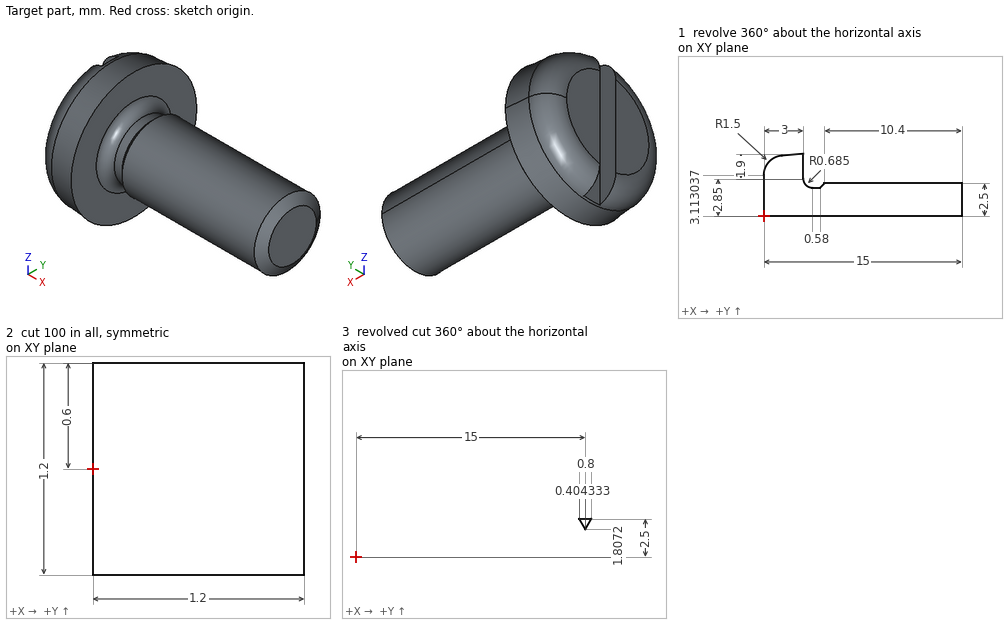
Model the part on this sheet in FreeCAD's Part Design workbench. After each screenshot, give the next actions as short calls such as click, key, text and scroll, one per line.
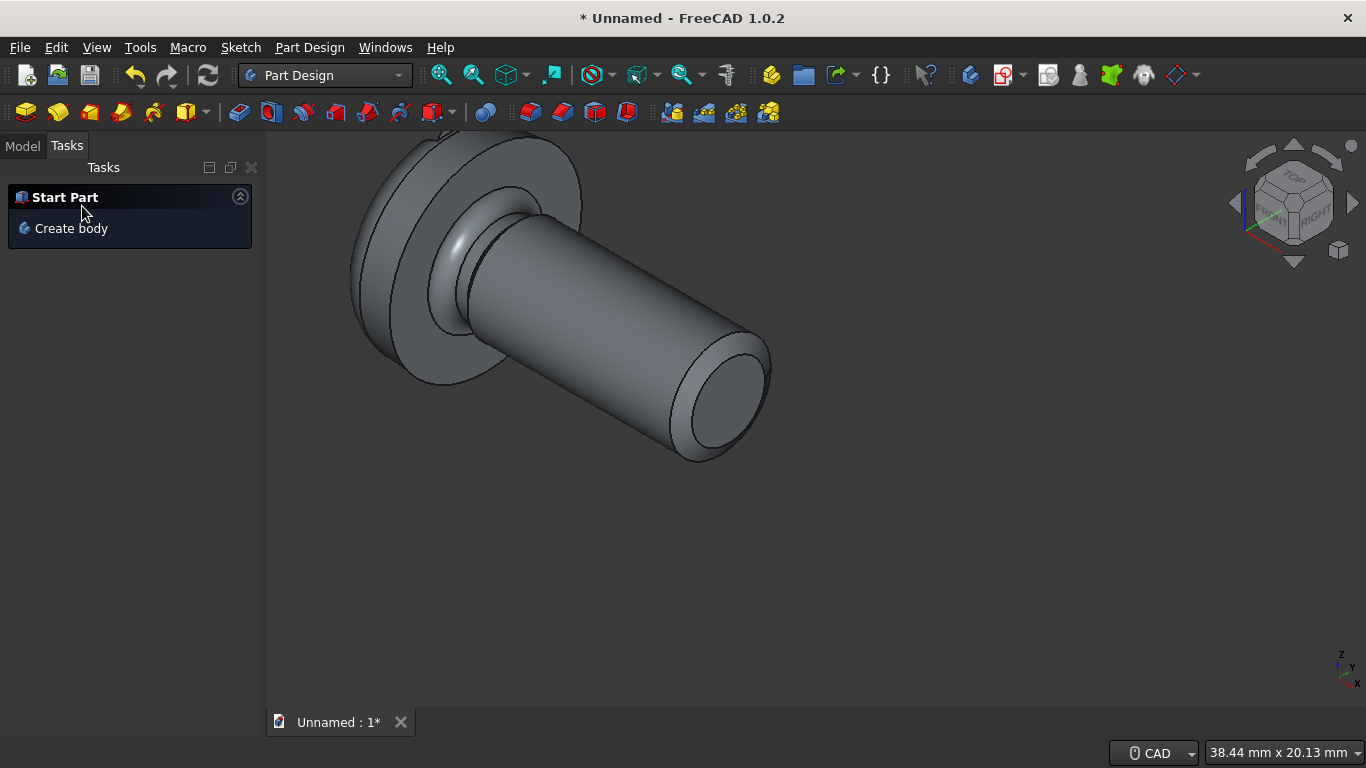
key(v)
key(f)